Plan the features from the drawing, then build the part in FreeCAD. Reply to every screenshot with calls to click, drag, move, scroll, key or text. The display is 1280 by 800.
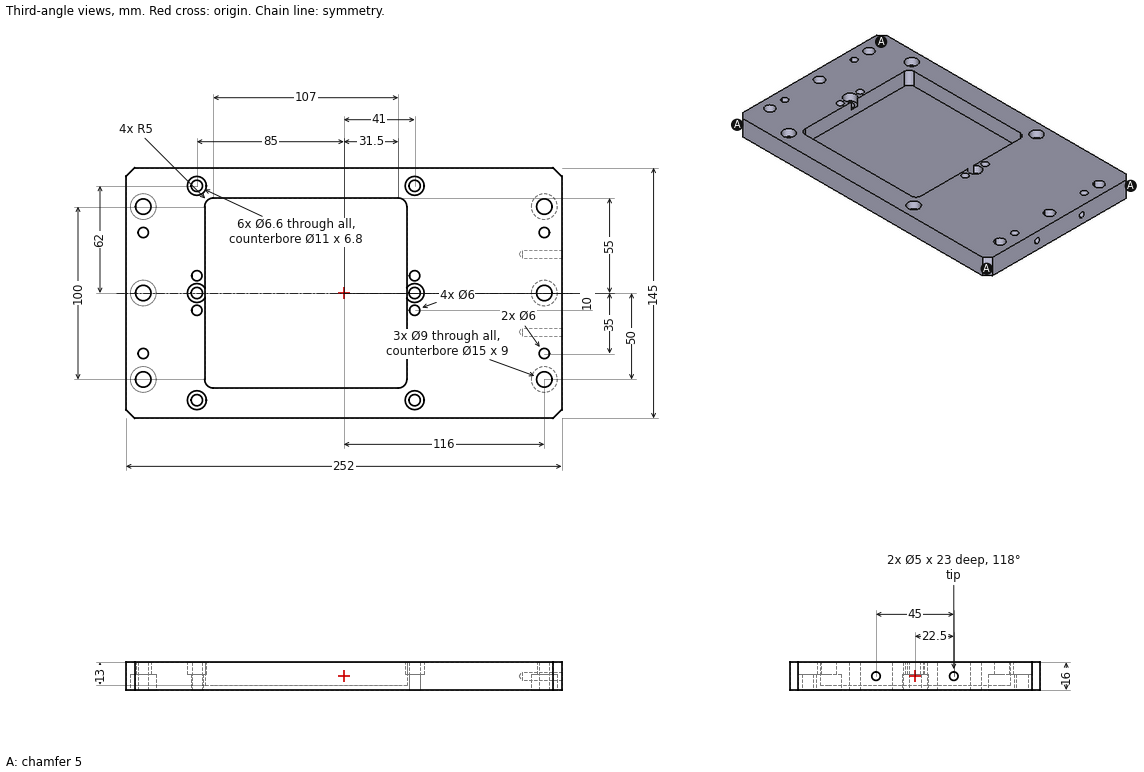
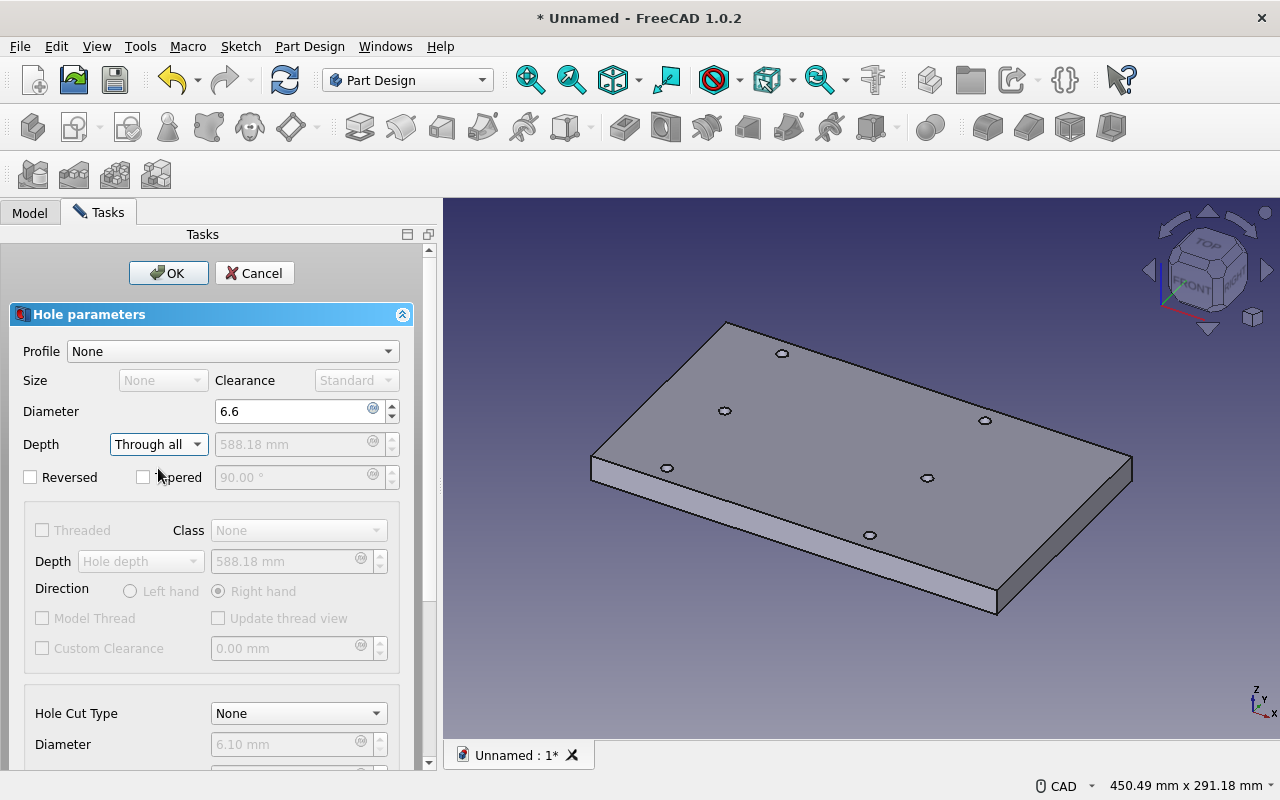
click(300, 714)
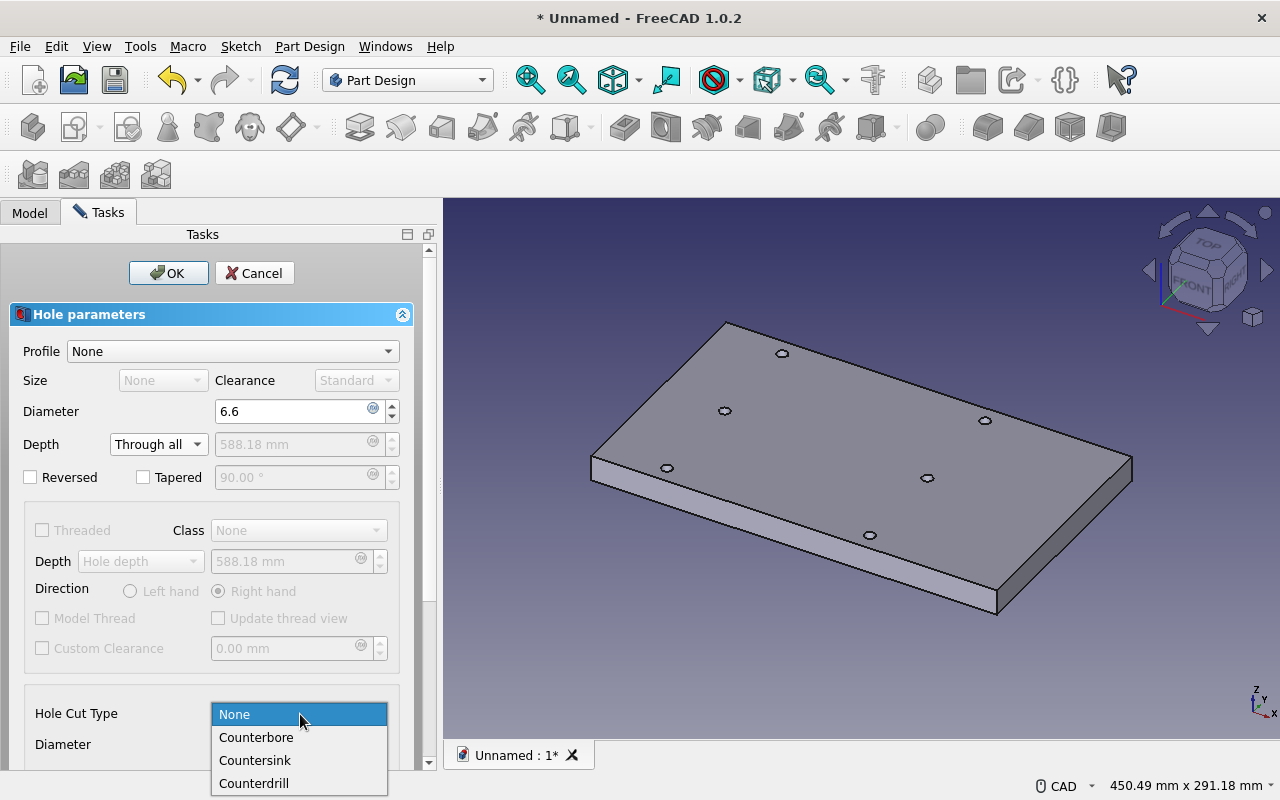
click(298, 738)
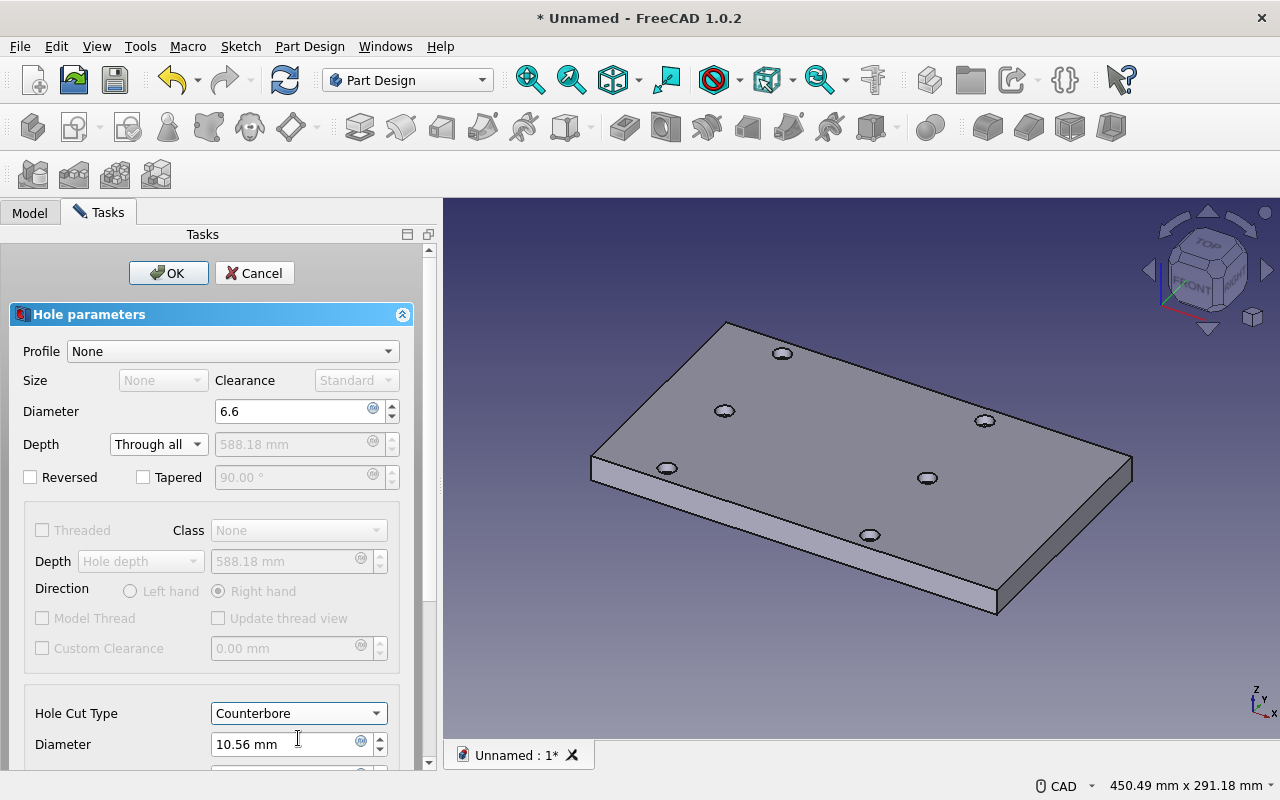
triple_click(292, 744)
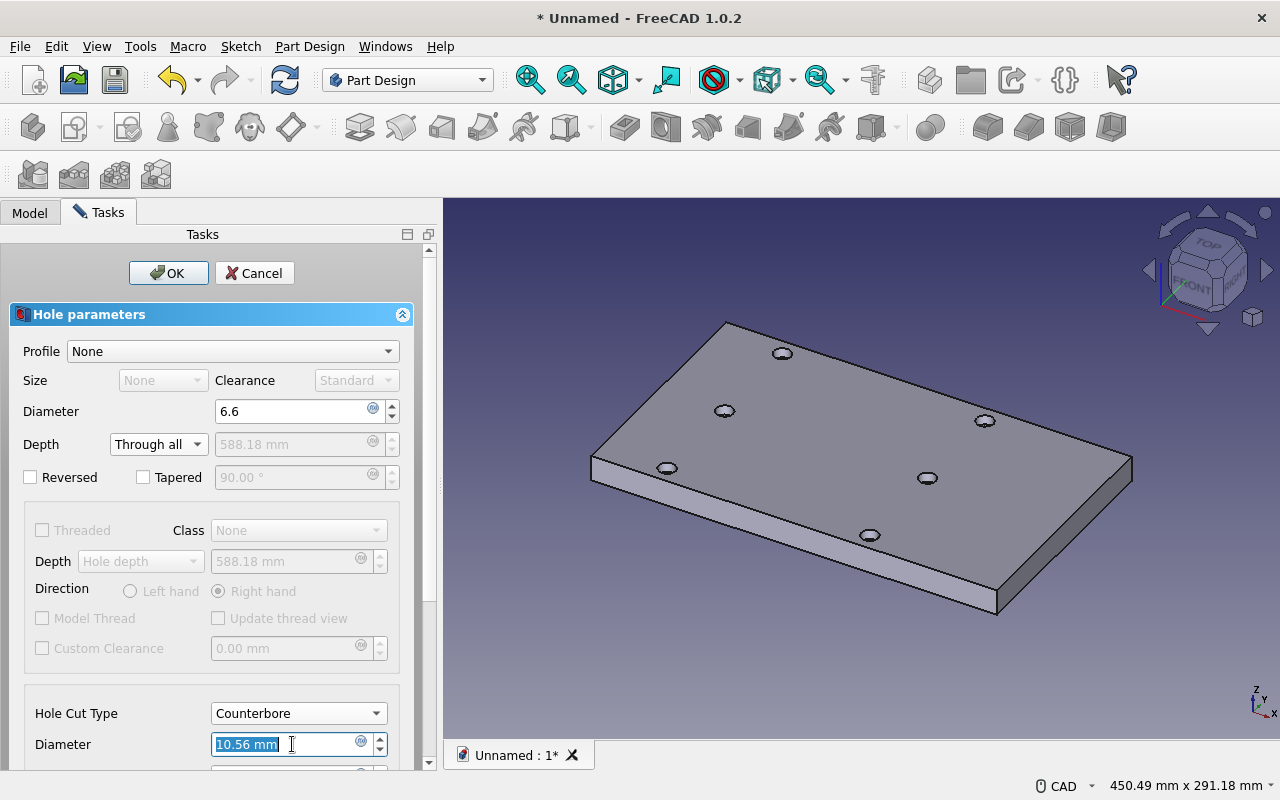
text(11)
key(Tab)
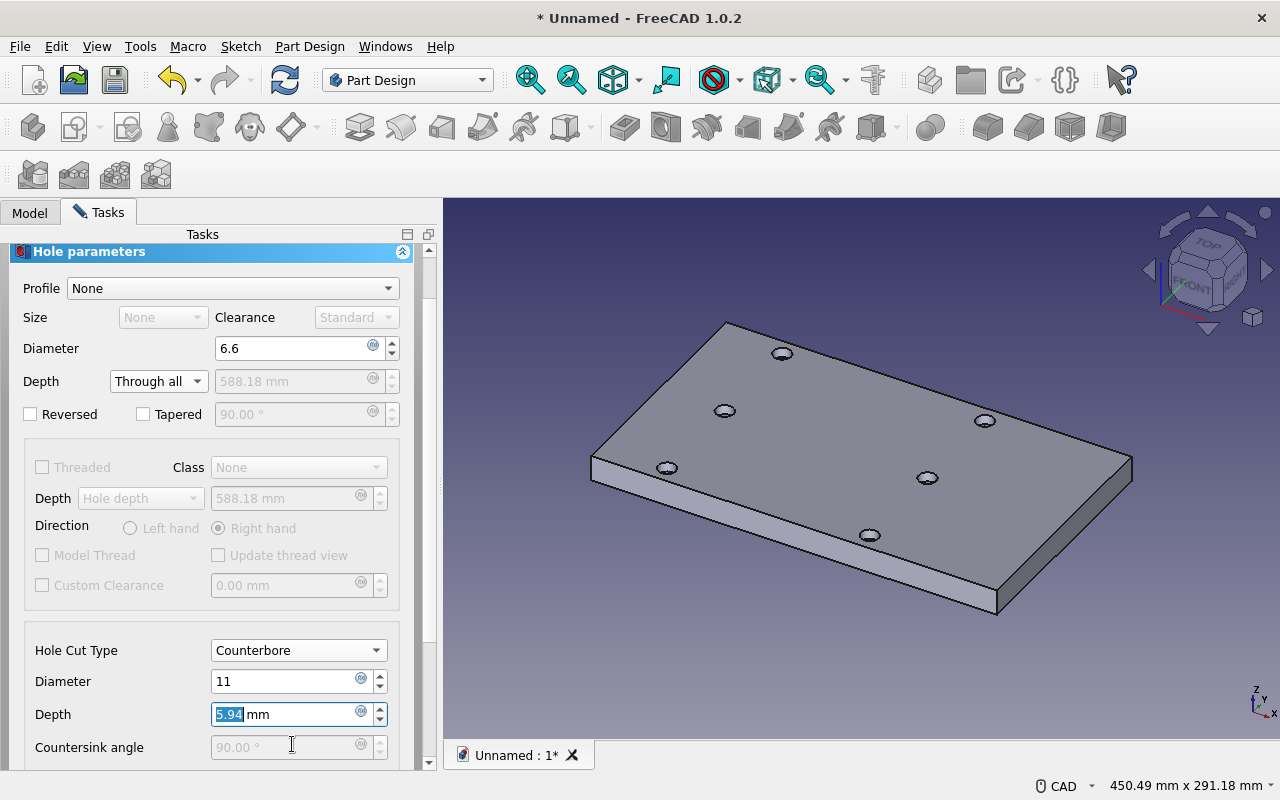
text(6.8)
key(Tab)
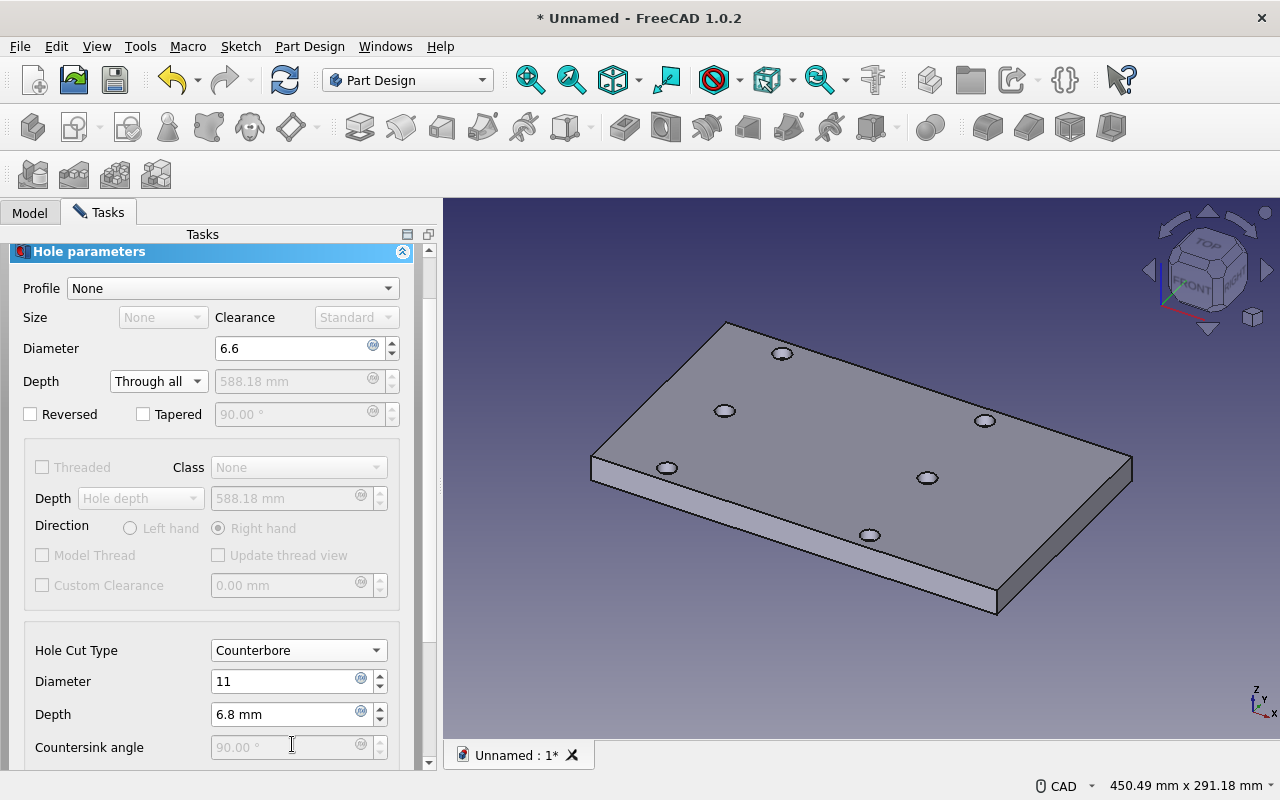
scroll(429, 507, up, 2)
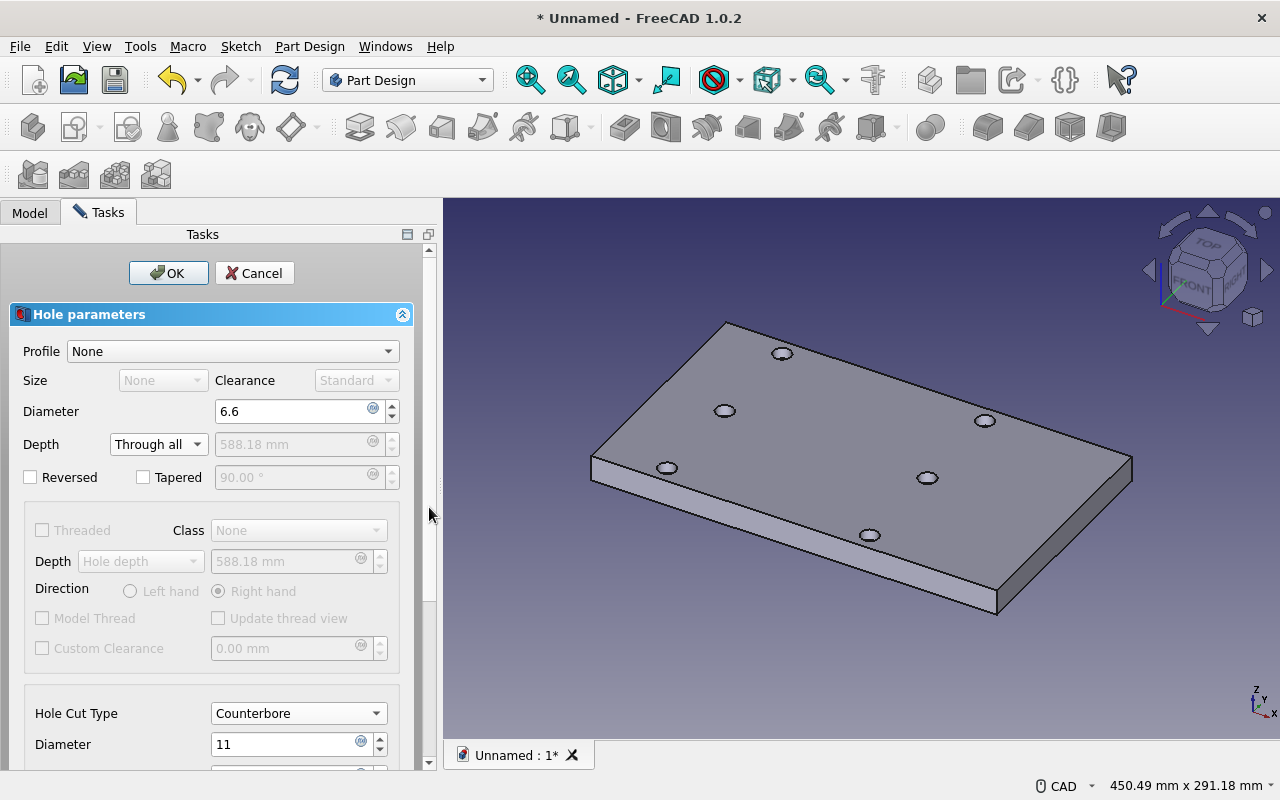
click(169, 273)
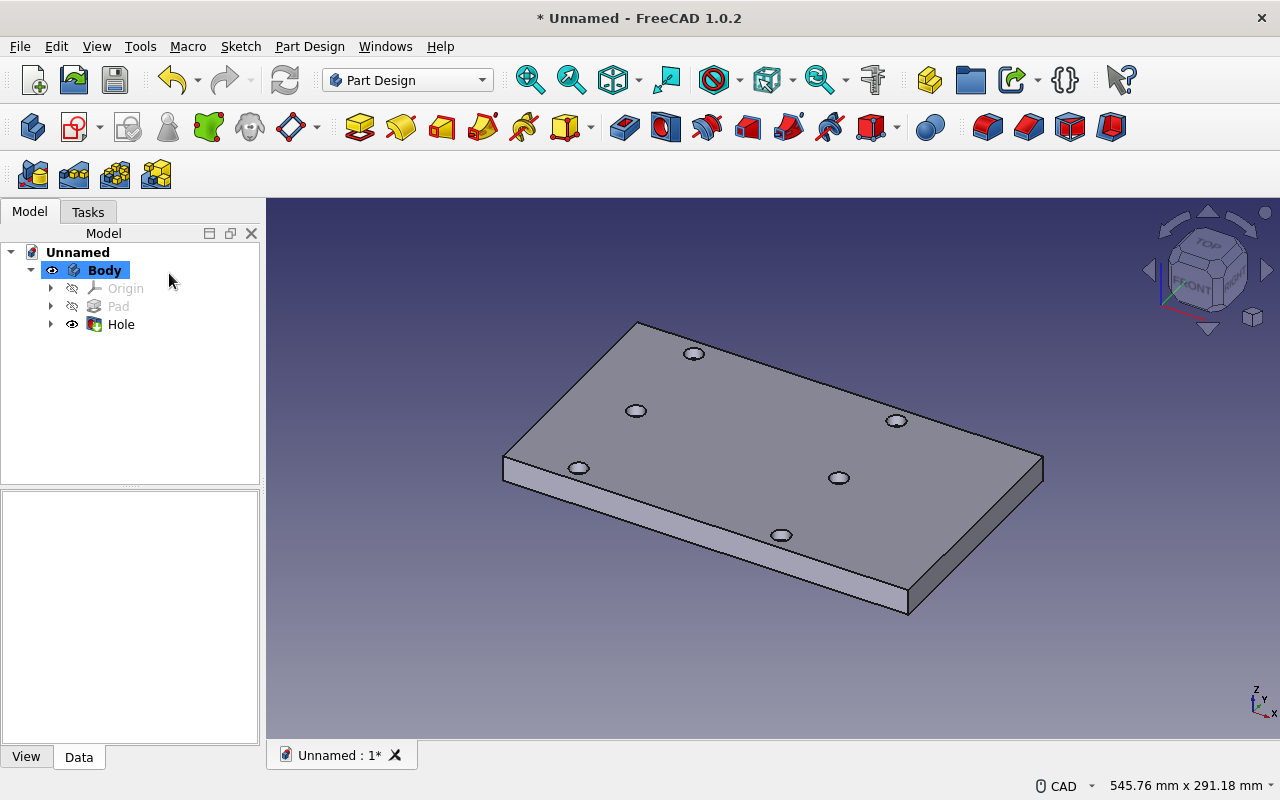
key(5)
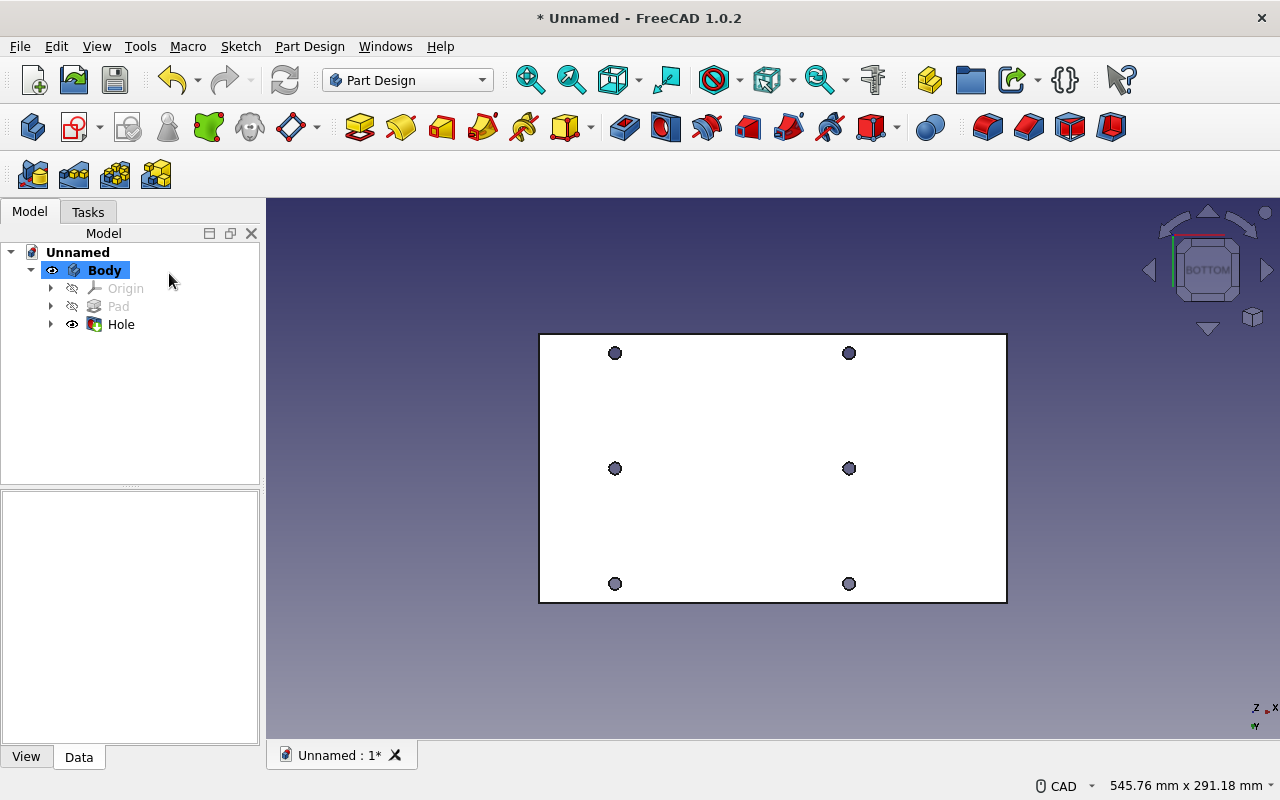
click(706, 429)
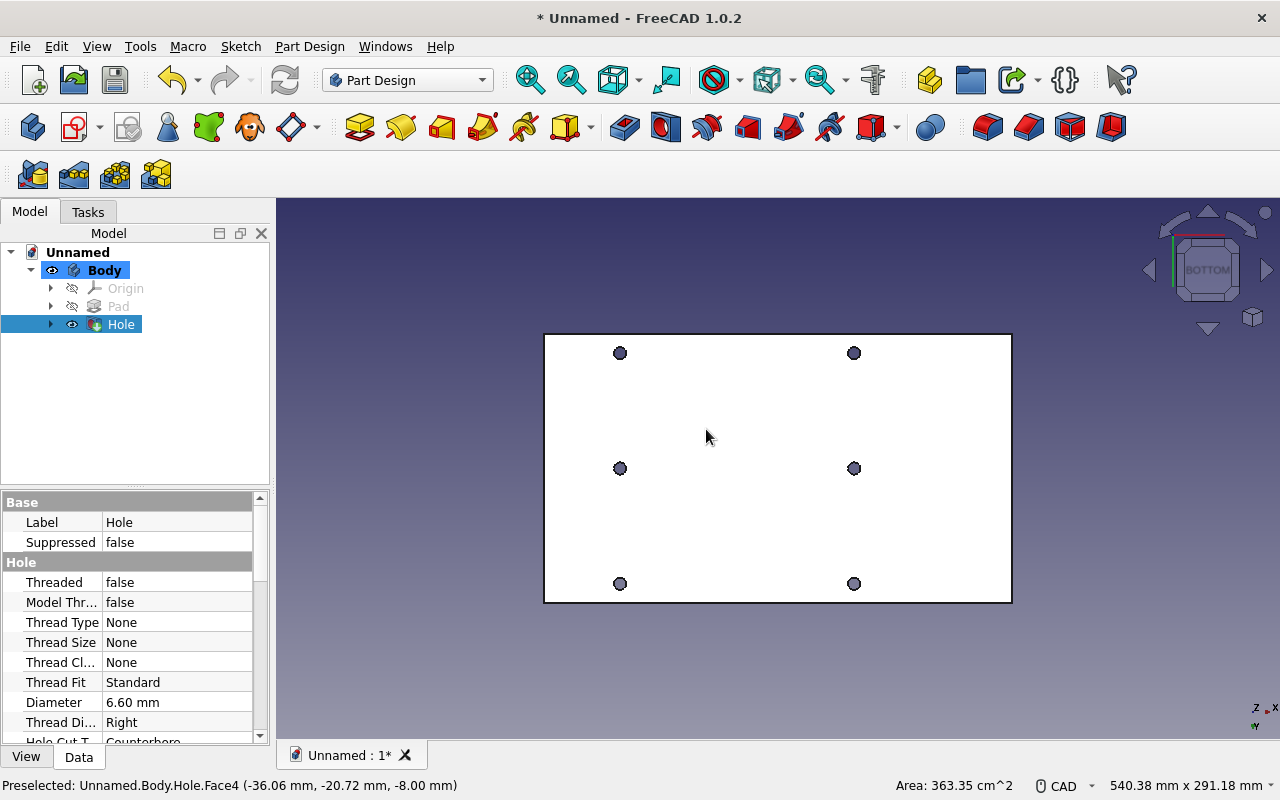
click(74, 128)